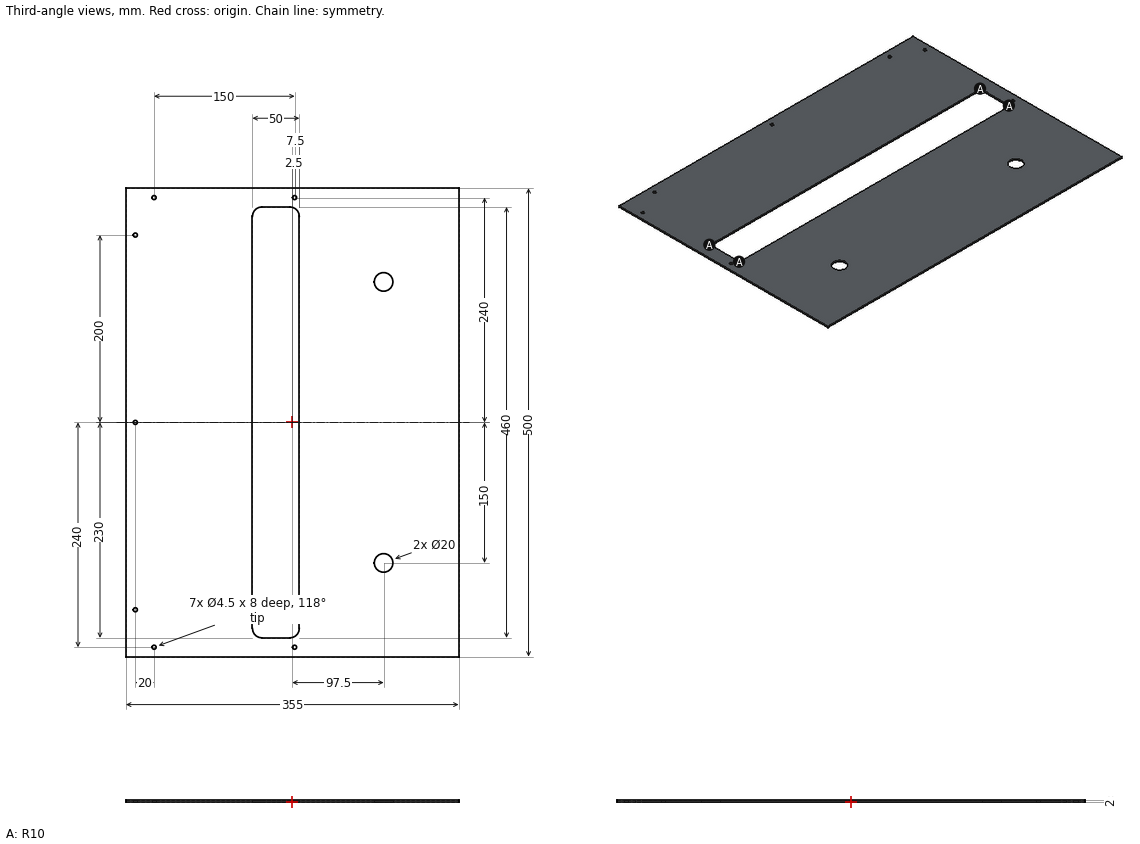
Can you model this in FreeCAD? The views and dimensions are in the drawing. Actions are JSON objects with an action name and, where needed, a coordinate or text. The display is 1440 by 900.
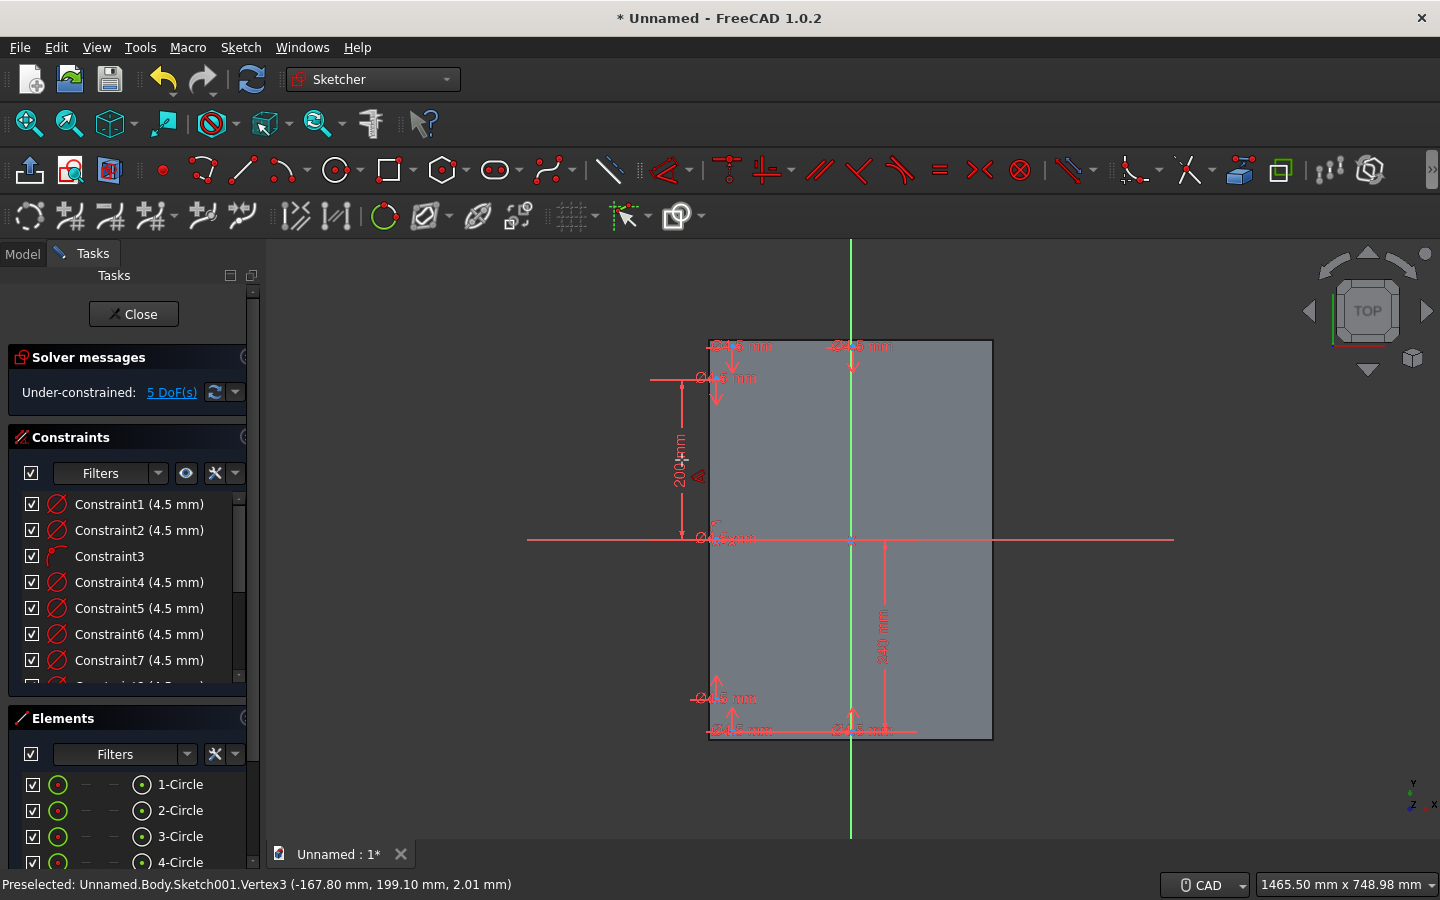
{"action": "scroll", "coordinate": [853, 348], "scroll_direction": "up", "scroll_amount": 15}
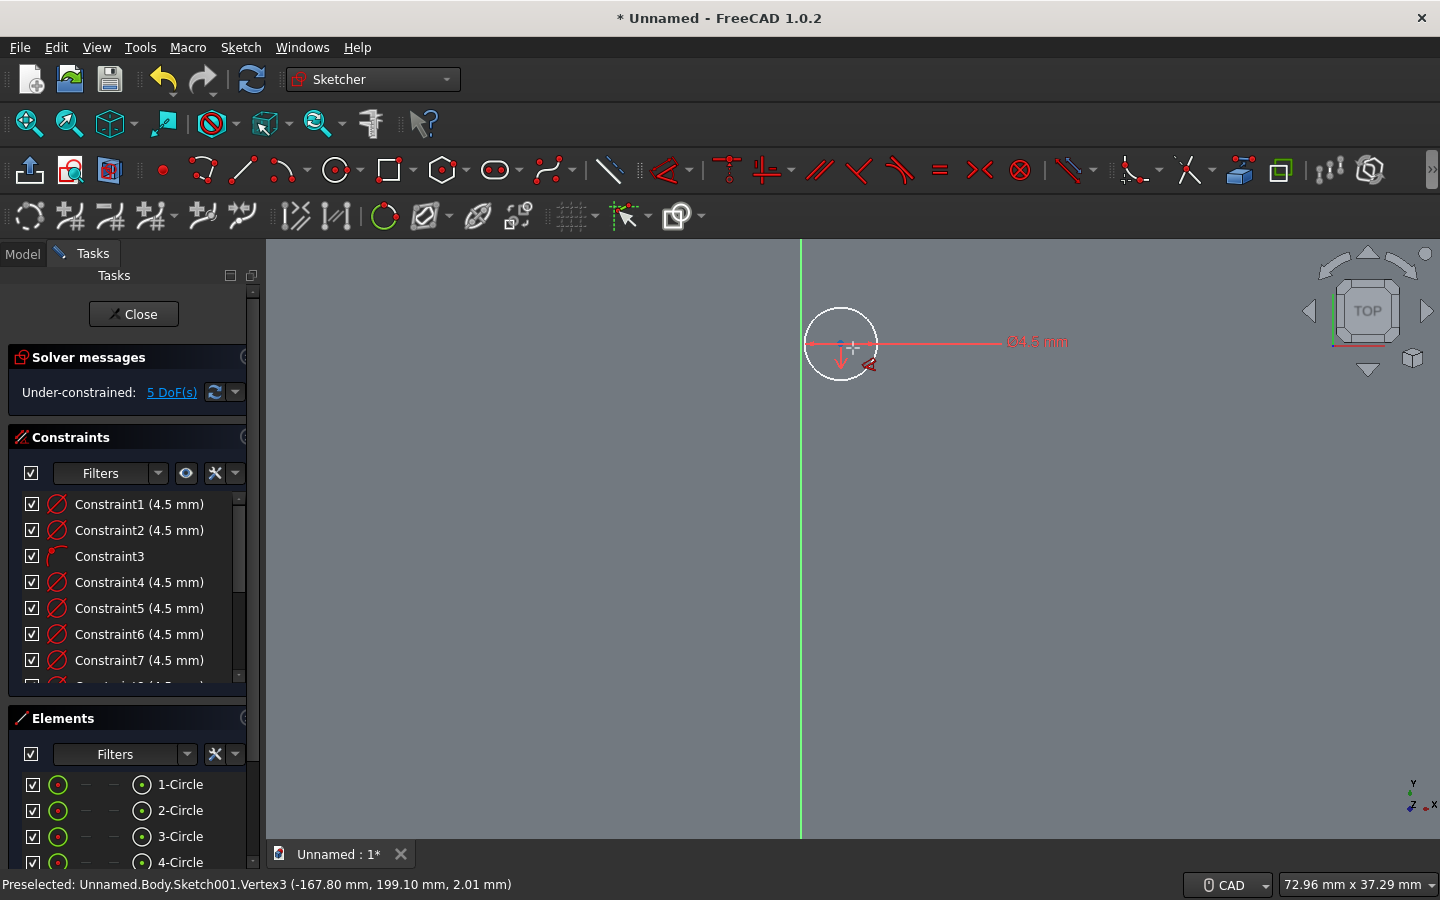
{"action": "left_click", "coordinate": [841, 344]}
{"action": "left_click", "coordinate": [821, 286]}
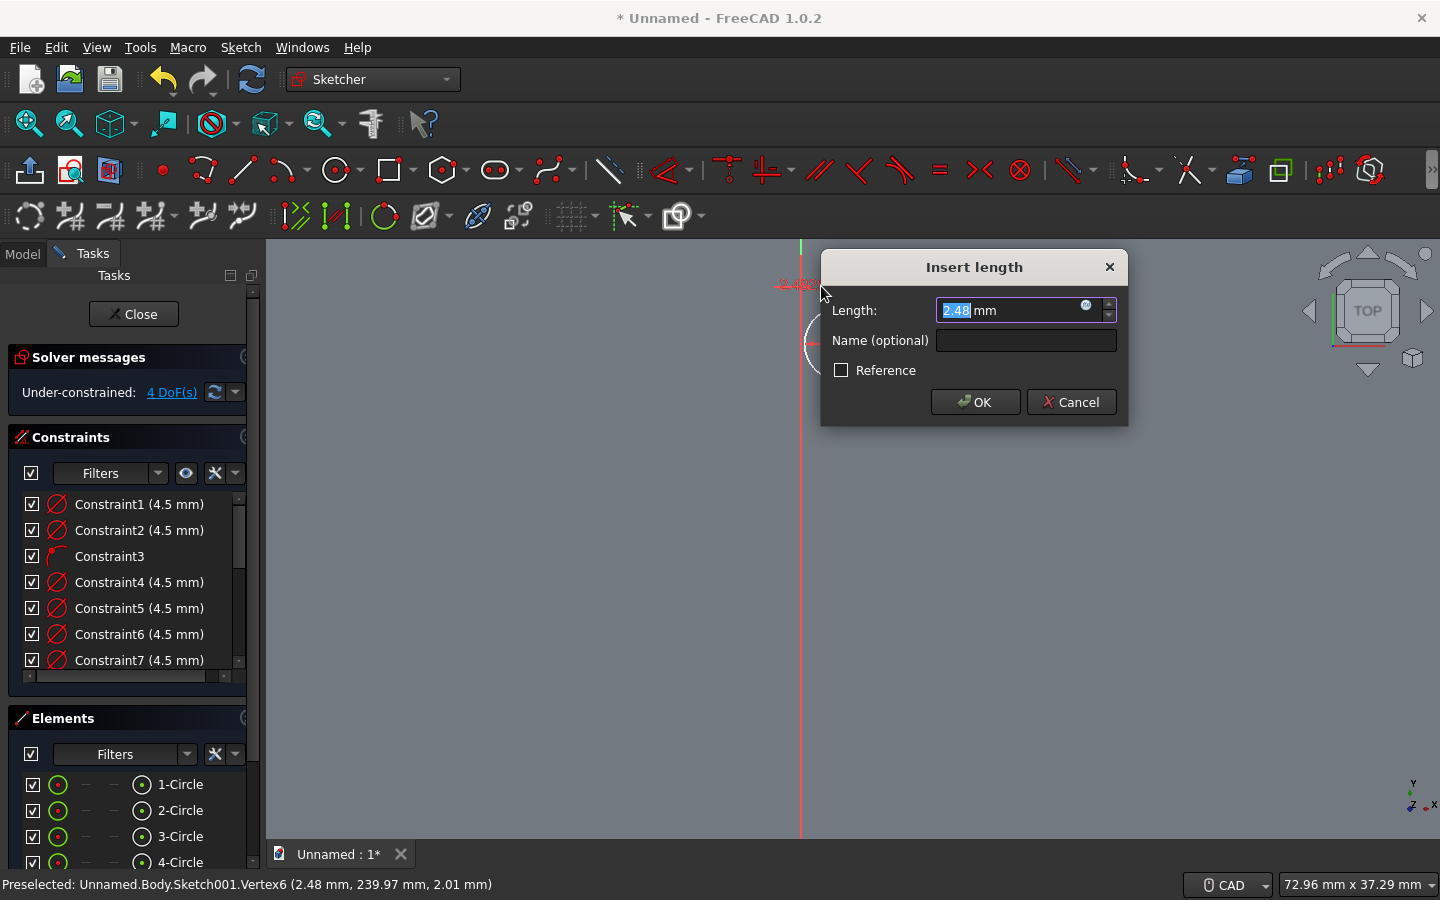
{"action": "type", "text": "2.5"}
{"action": "key", "text": "Return"}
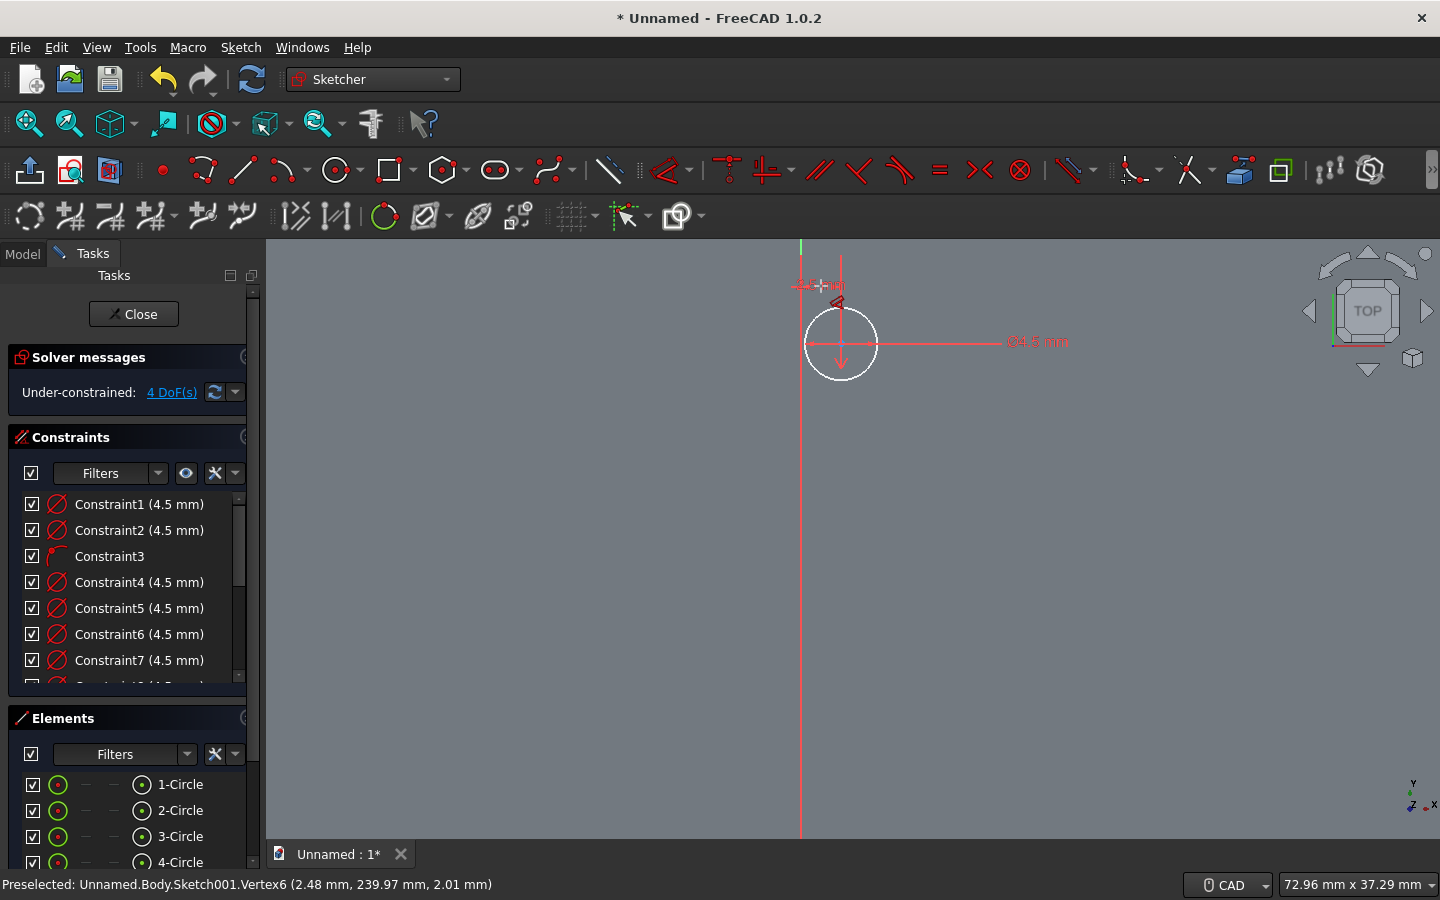
{"action": "scroll", "coordinate": [853, 347], "scroll_direction": "down", "scroll_amount": 15}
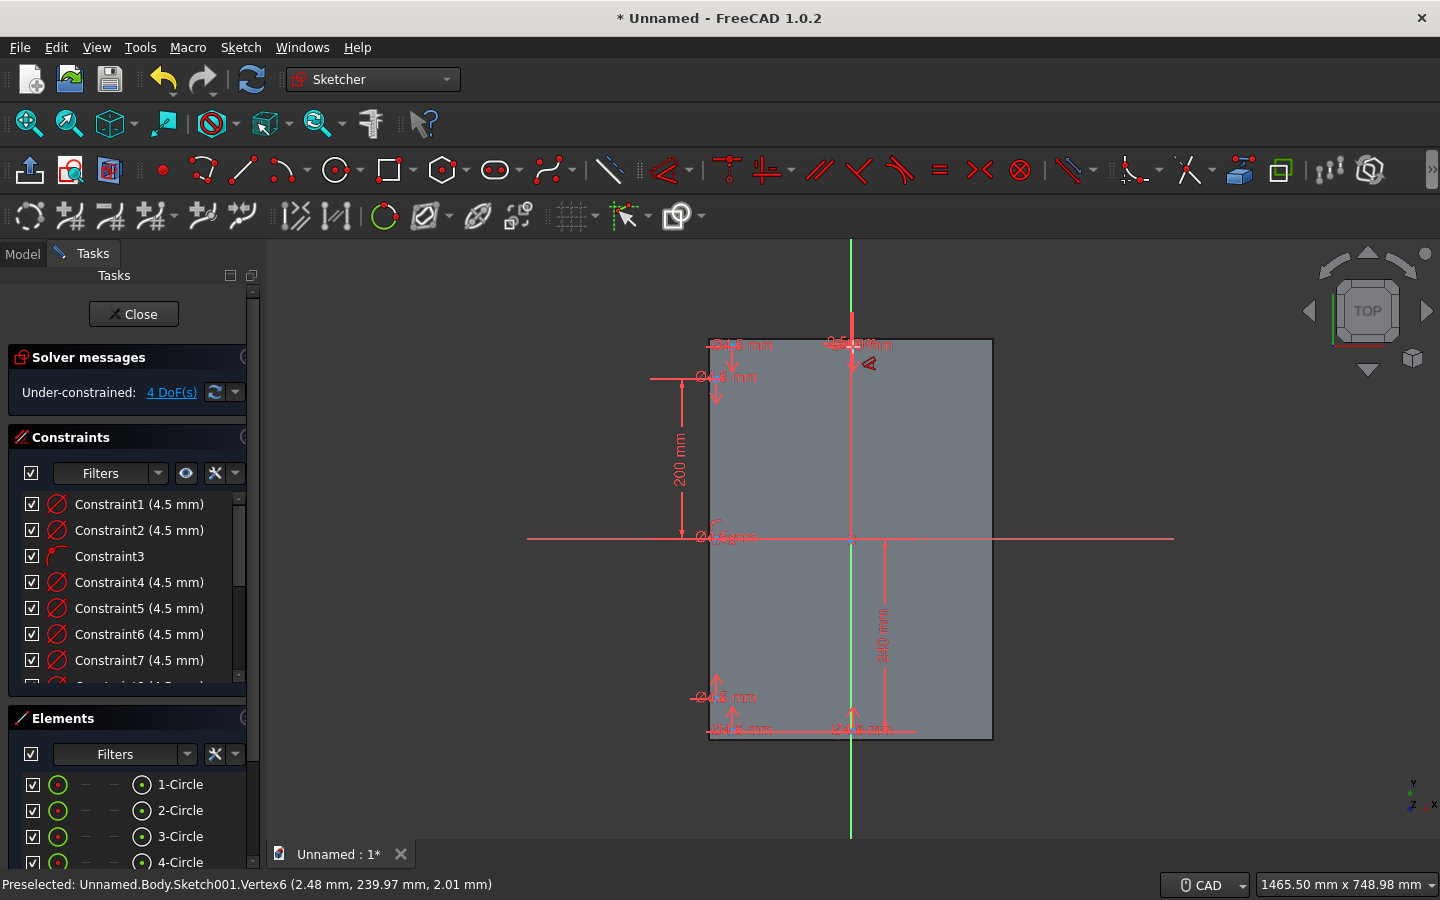
{"action": "left_click", "coordinate": [853, 347]}
{"action": "left_click", "coordinate": [887, 443]}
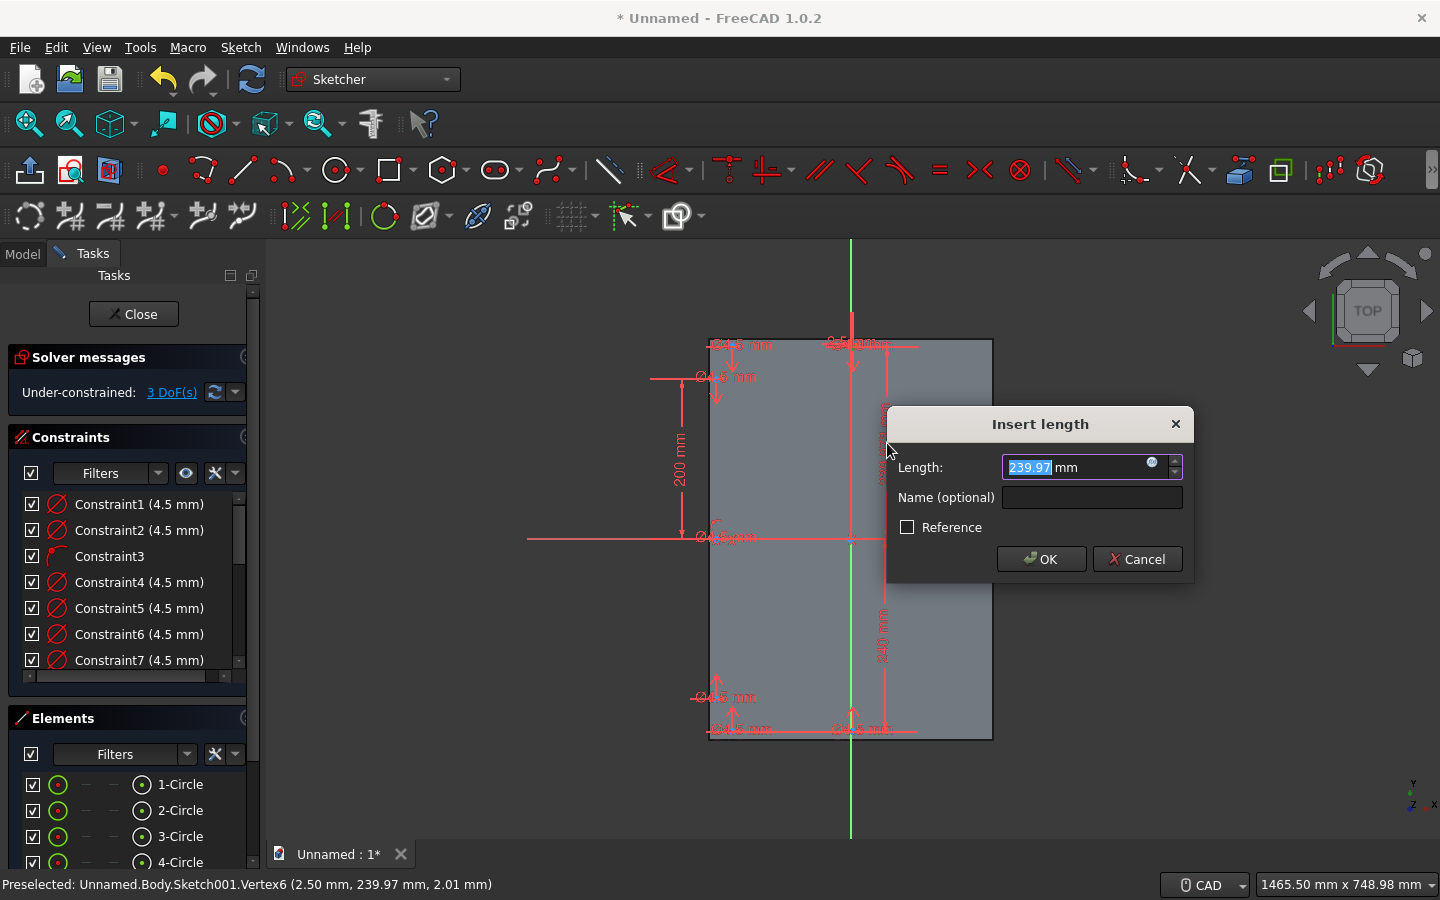
{"action": "type", "text": "240"}
{"action": "key", "text": "Return"}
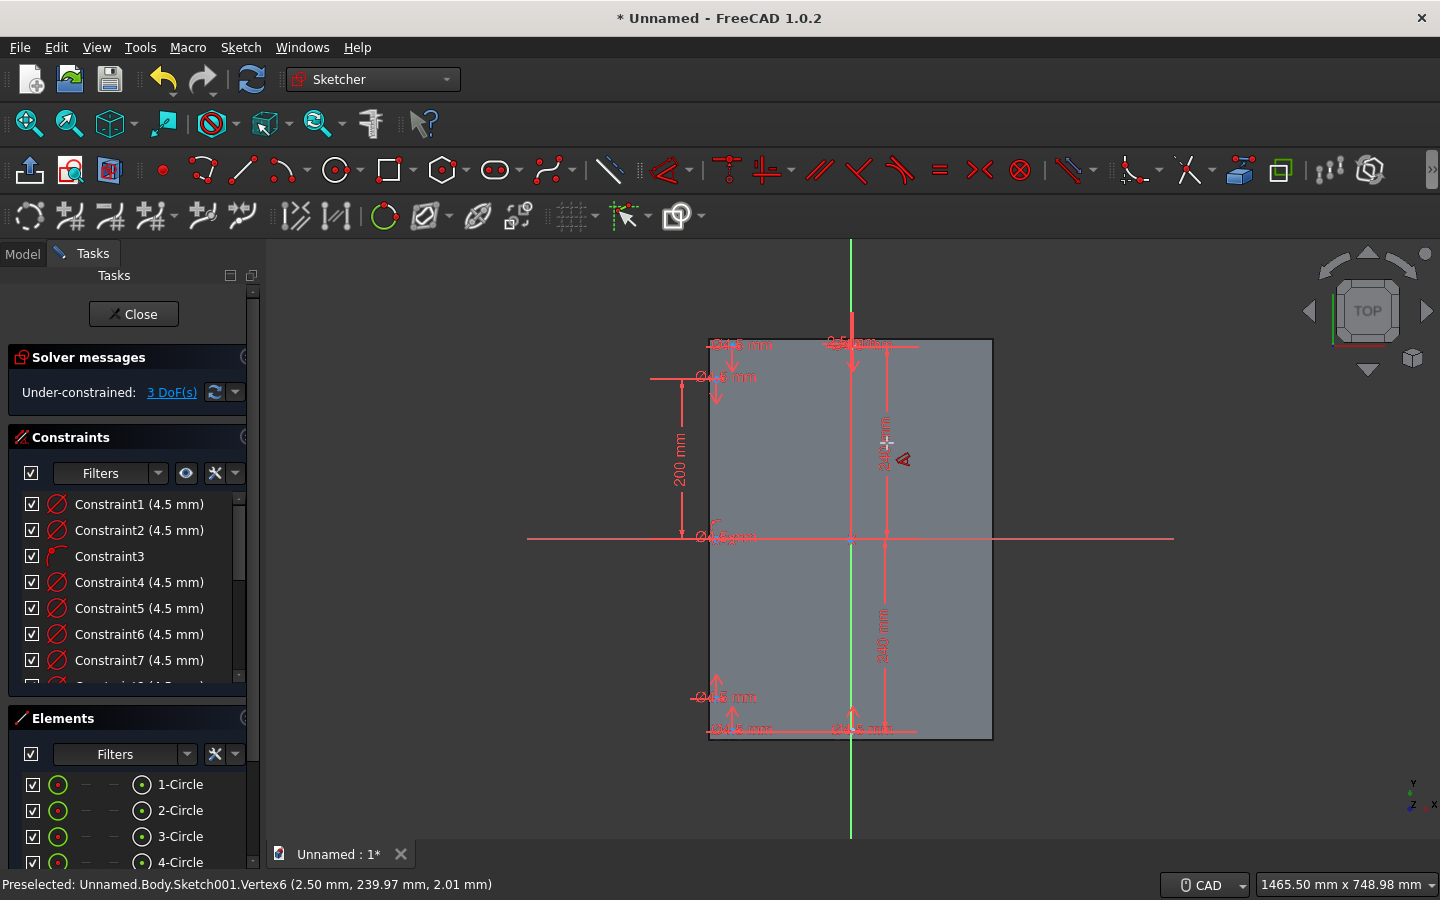
{"action": "scroll", "coordinate": [732, 732], "scroll_direction": "up", "scroll_amount": 5}